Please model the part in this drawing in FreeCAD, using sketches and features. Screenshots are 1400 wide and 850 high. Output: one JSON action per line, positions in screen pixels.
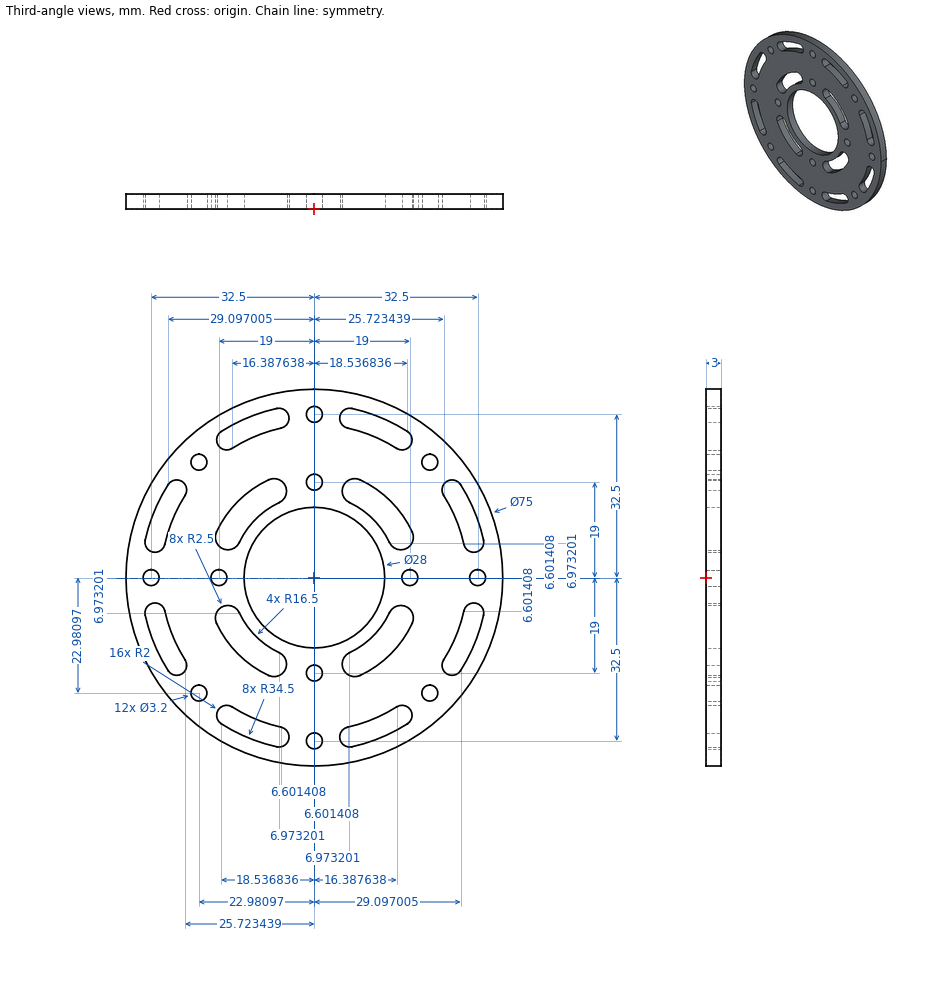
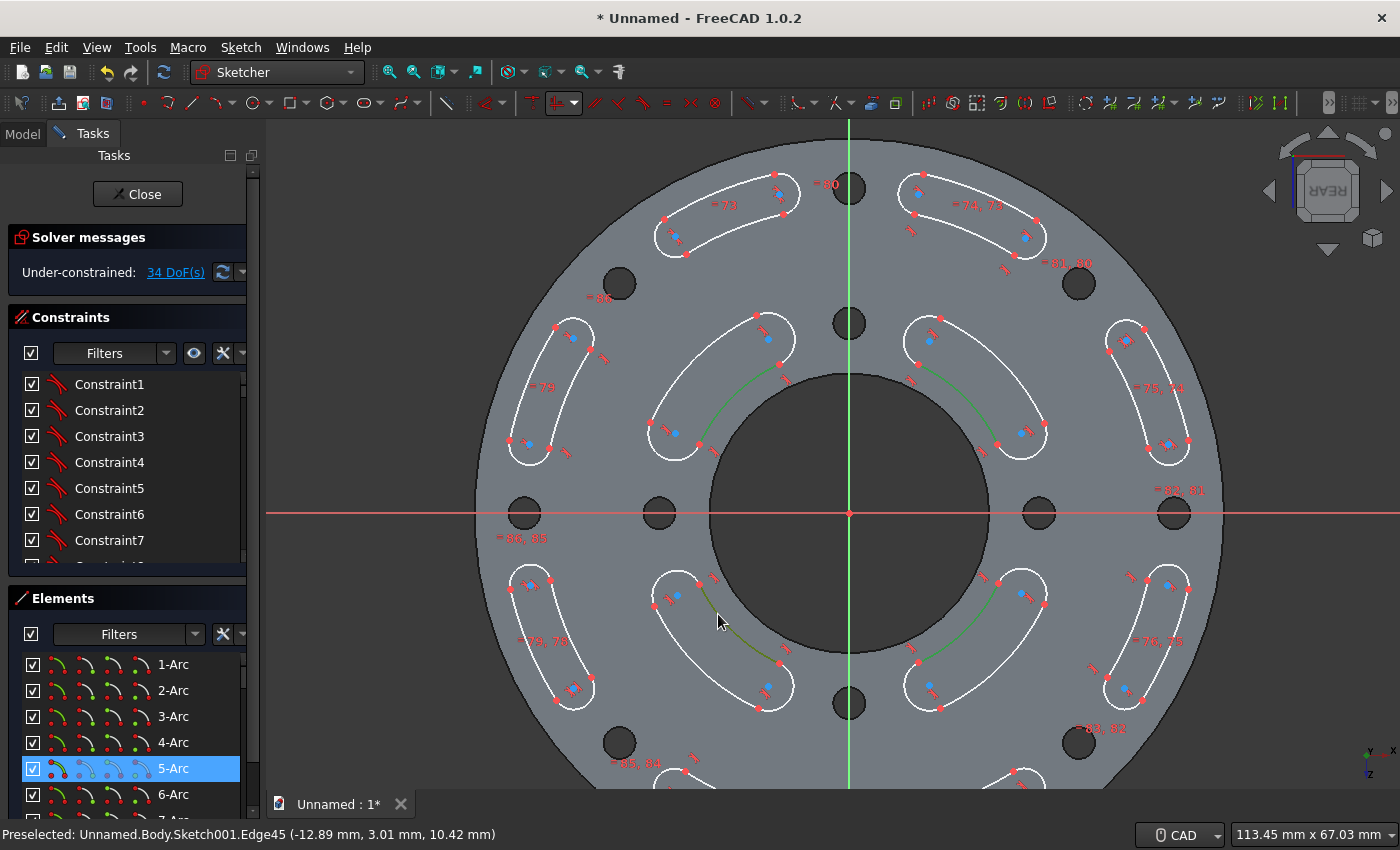
{"action": "left_click", "coordinate": [668, 104]}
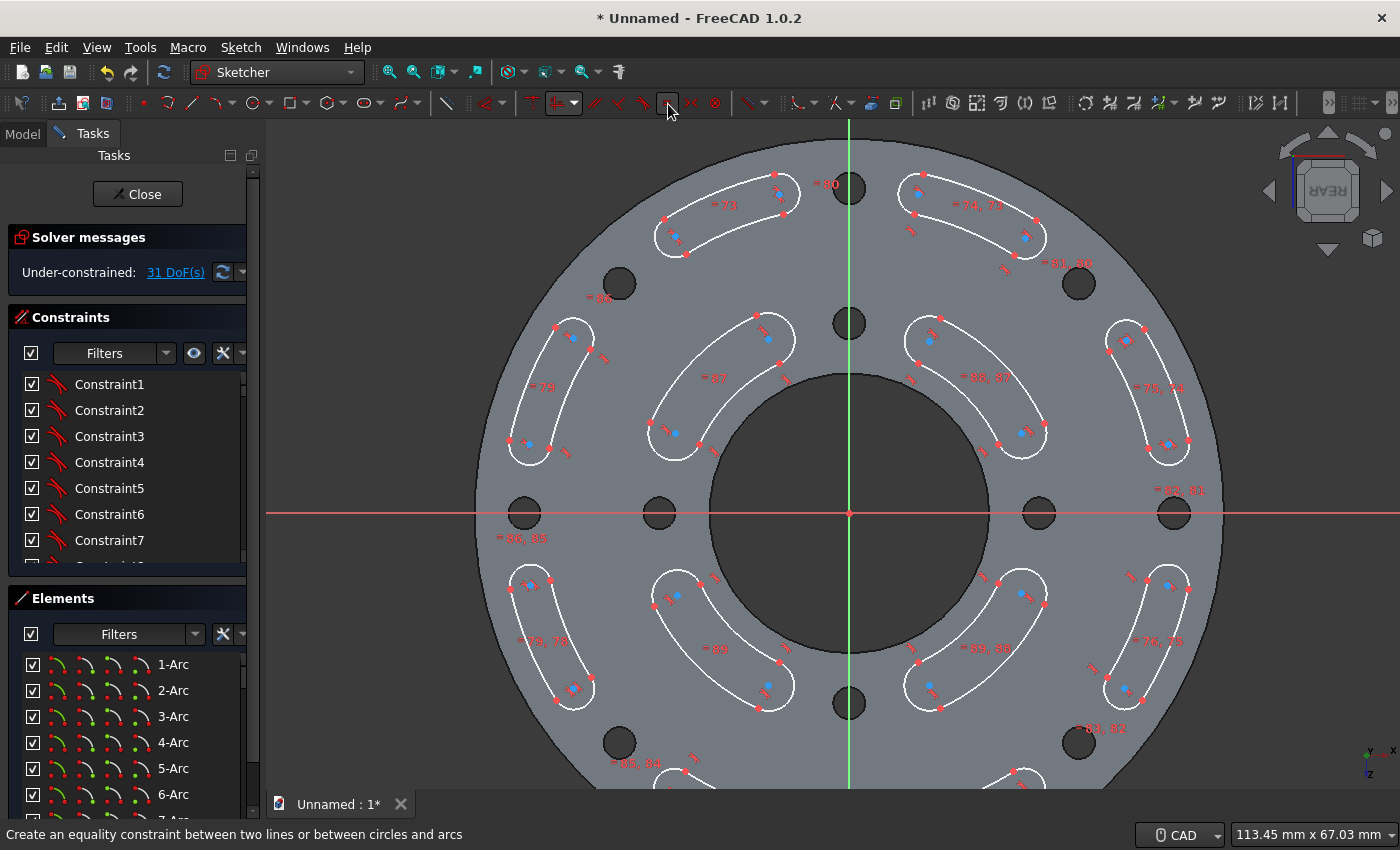
{"action": "left_click", "coordinate": [794, 345]}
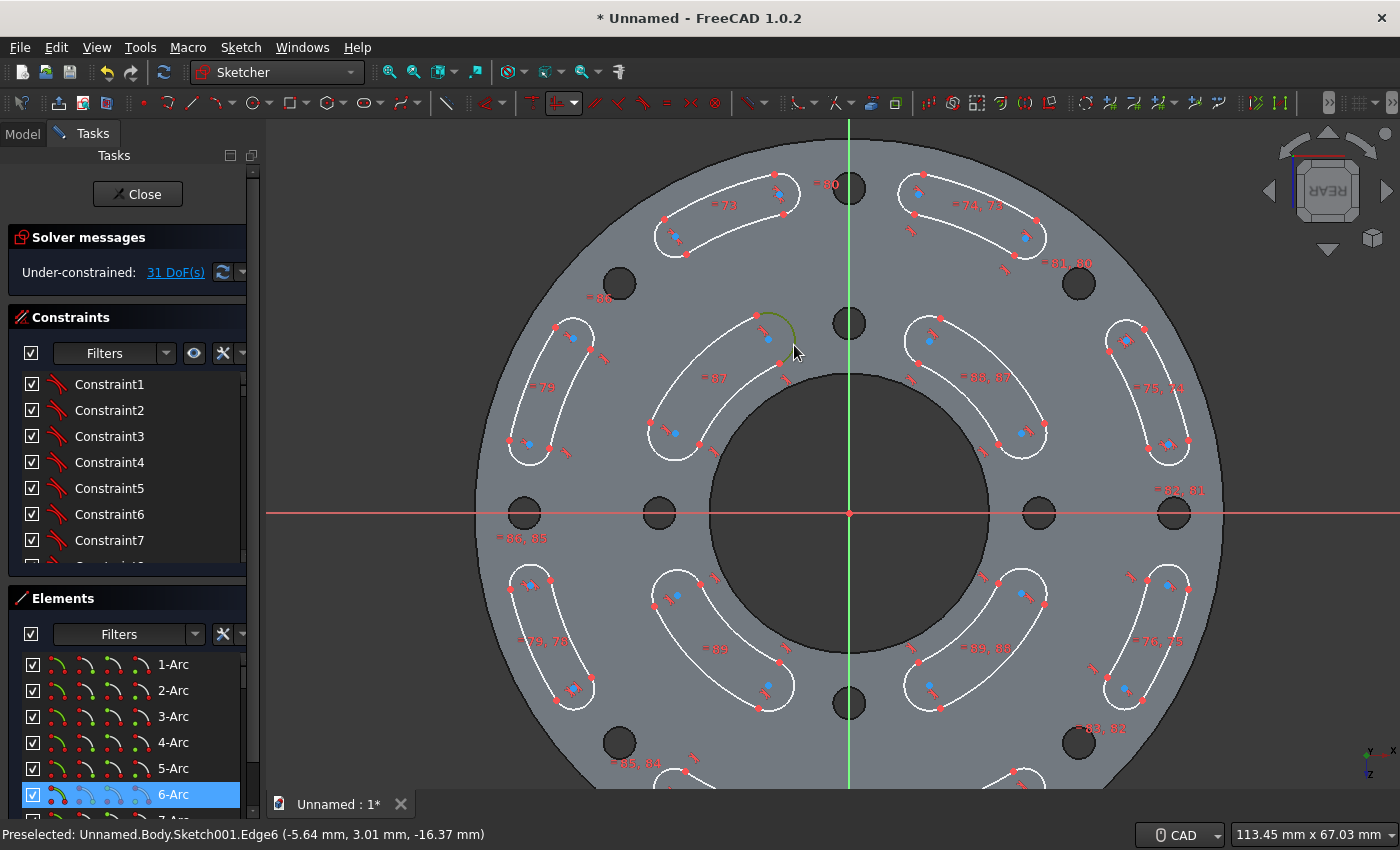
{"action": "left_click", "coordinate": [1017, 458]}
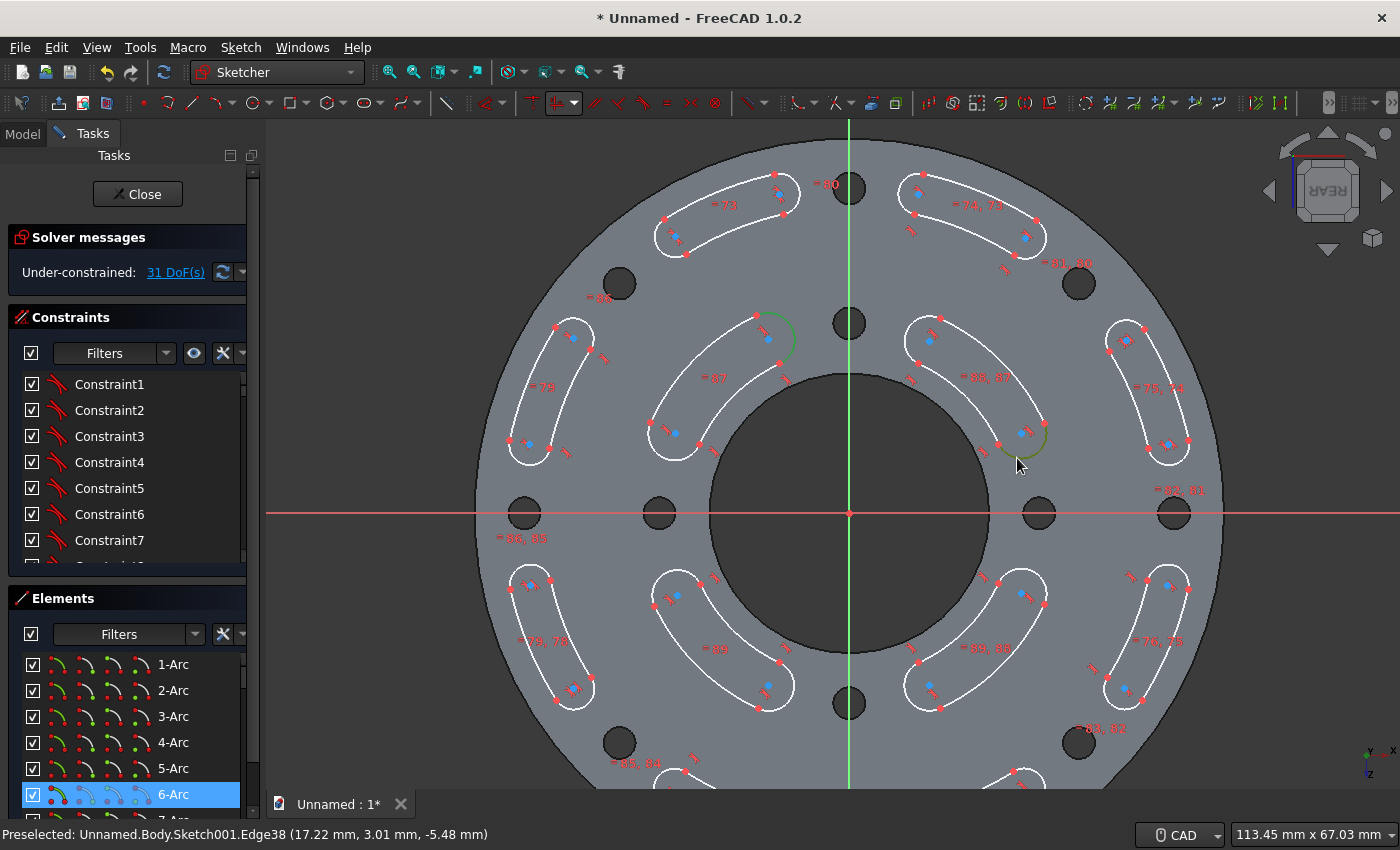
{"action": "left_click", "coordinate": [905, 681]}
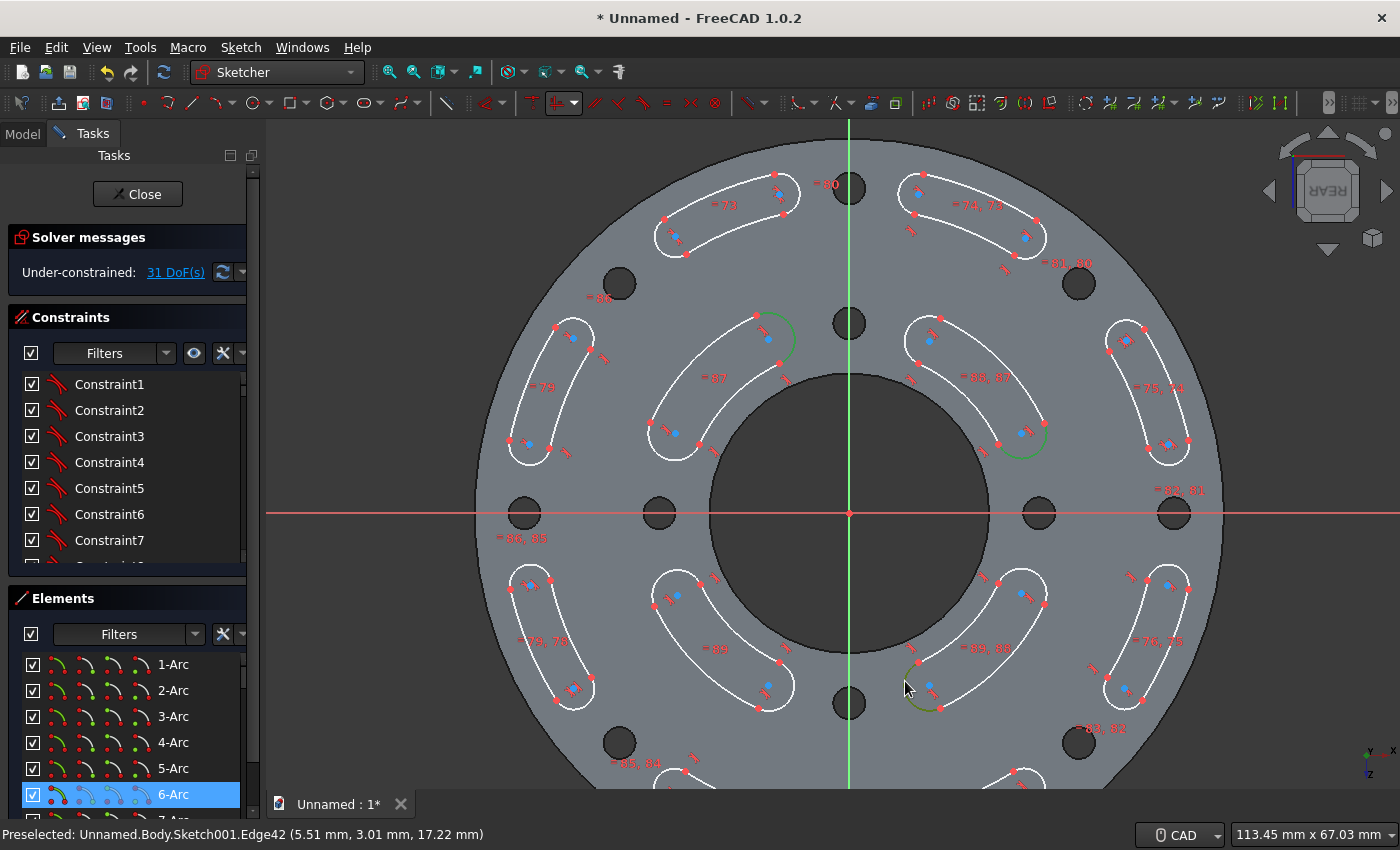
{"action": "left_click", "coordinate": [682, 570]}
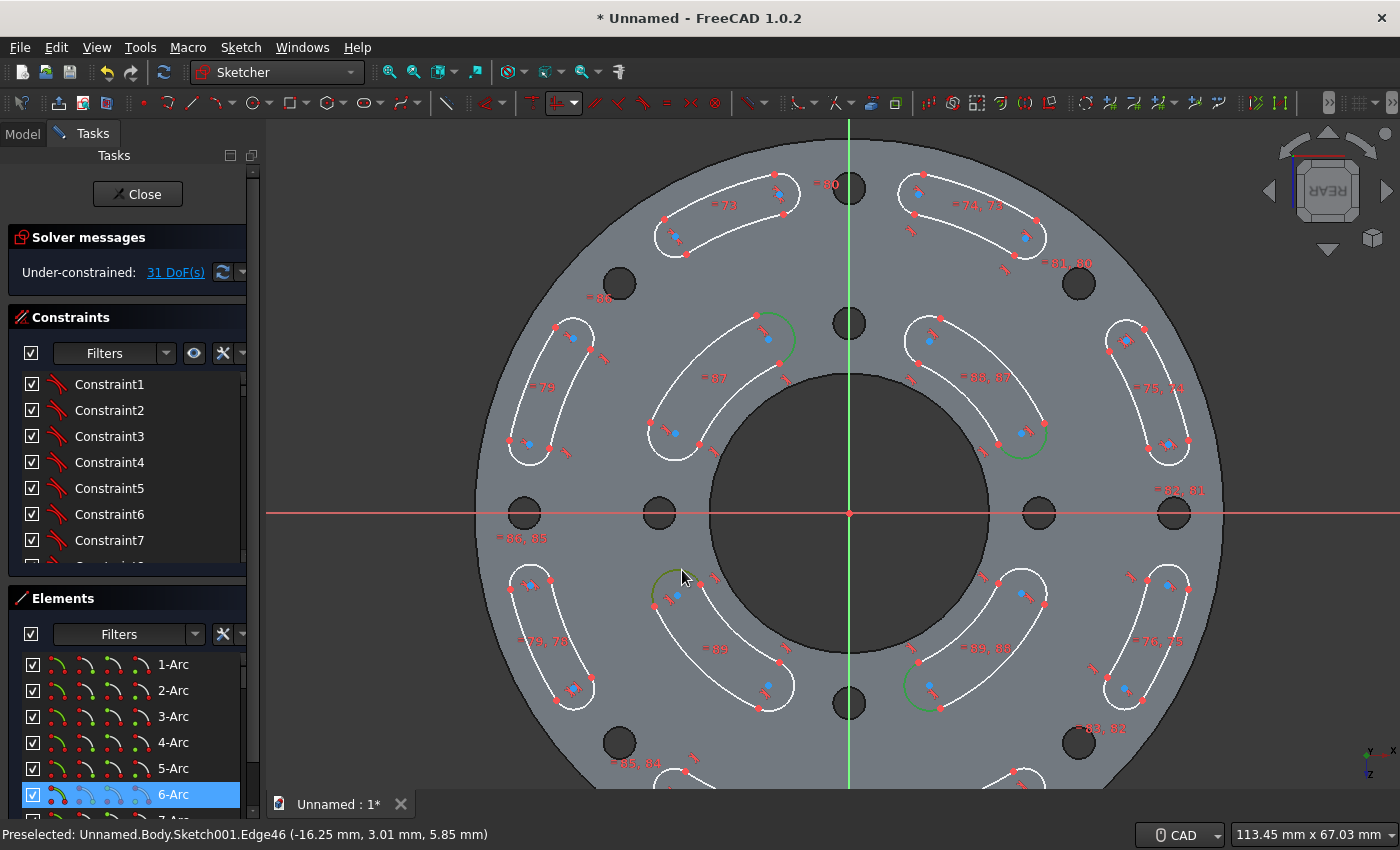
{"action": "left_click", "coordinate": [668, 104]}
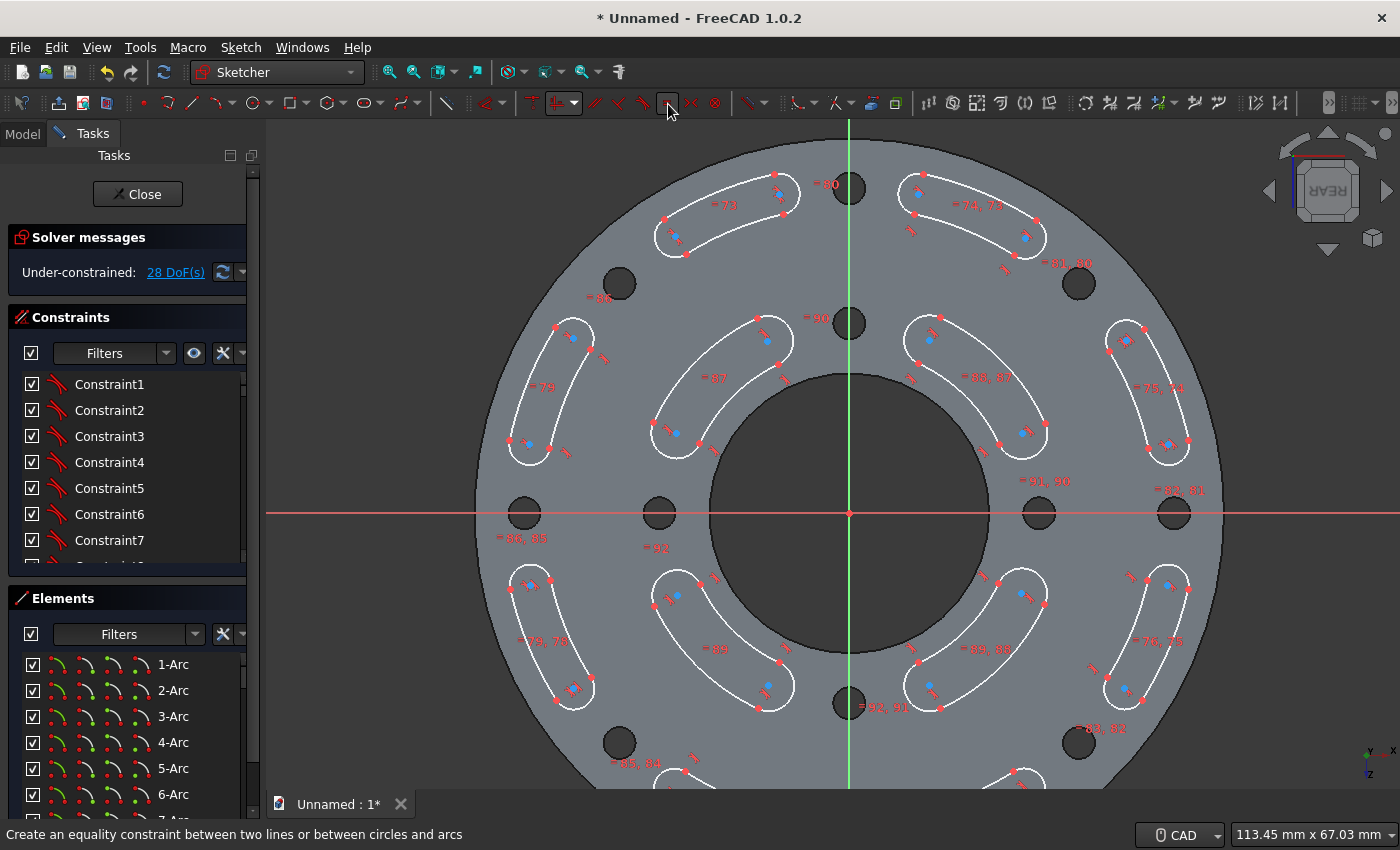
{"action": "left_click", "coordinate": [486, 104]}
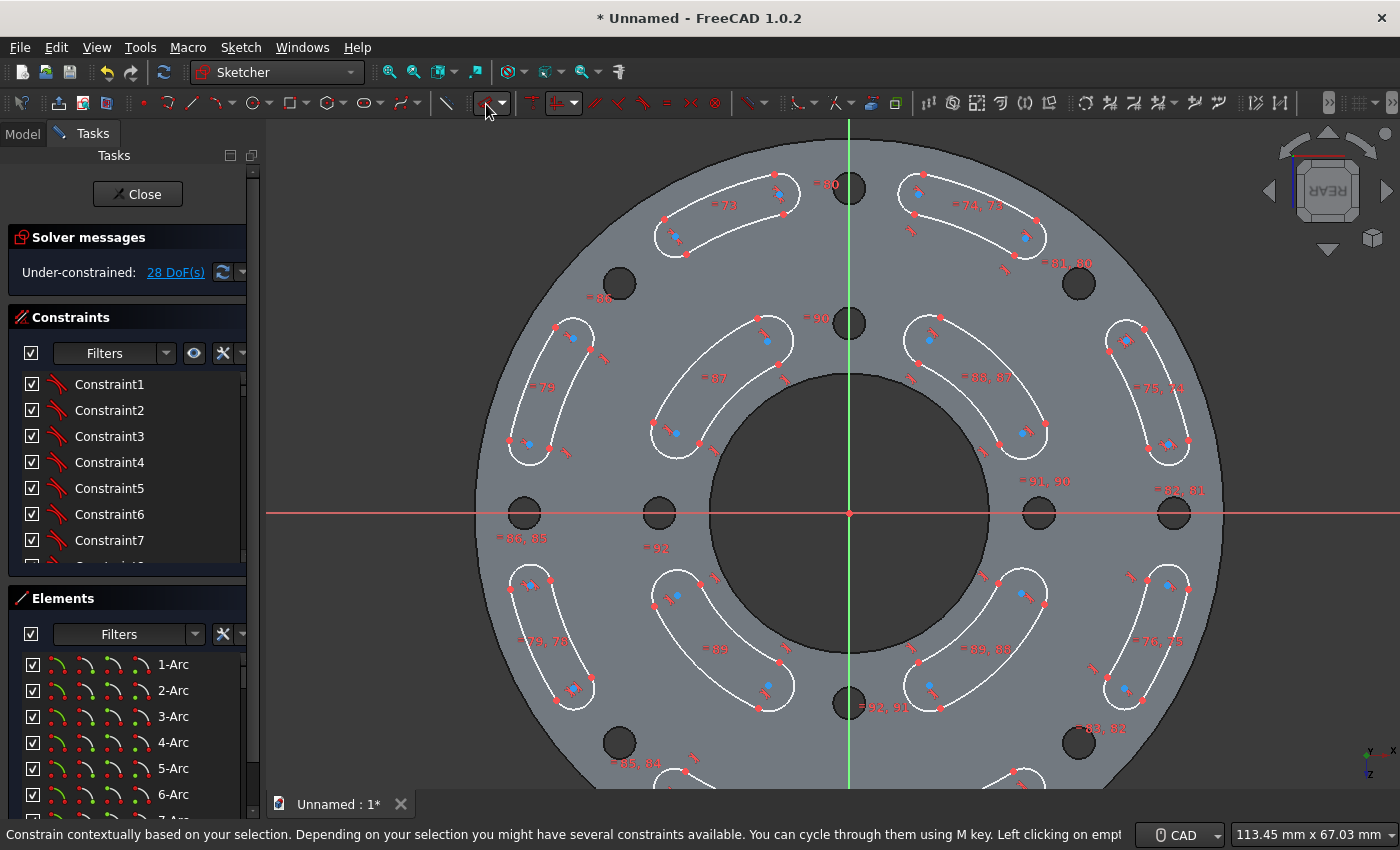
{"action": "scroll", "coordinate": [798, 202], "scroll_direction": "up", "scroll_amount": 4}